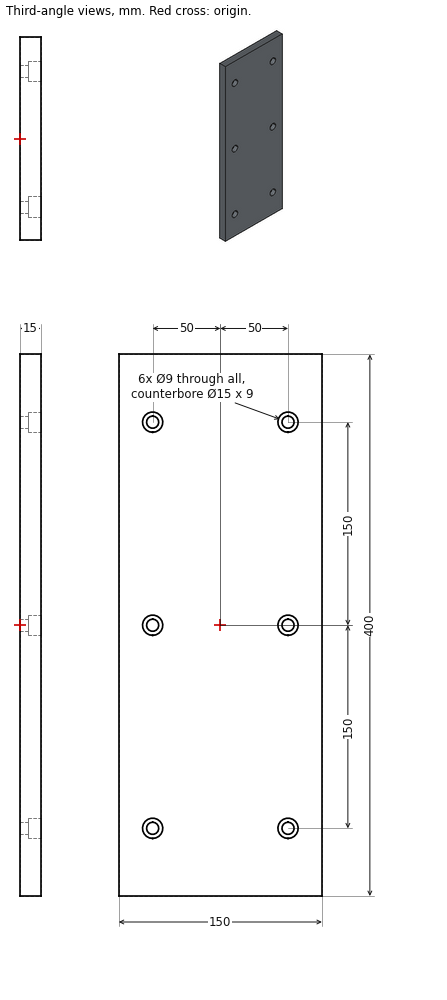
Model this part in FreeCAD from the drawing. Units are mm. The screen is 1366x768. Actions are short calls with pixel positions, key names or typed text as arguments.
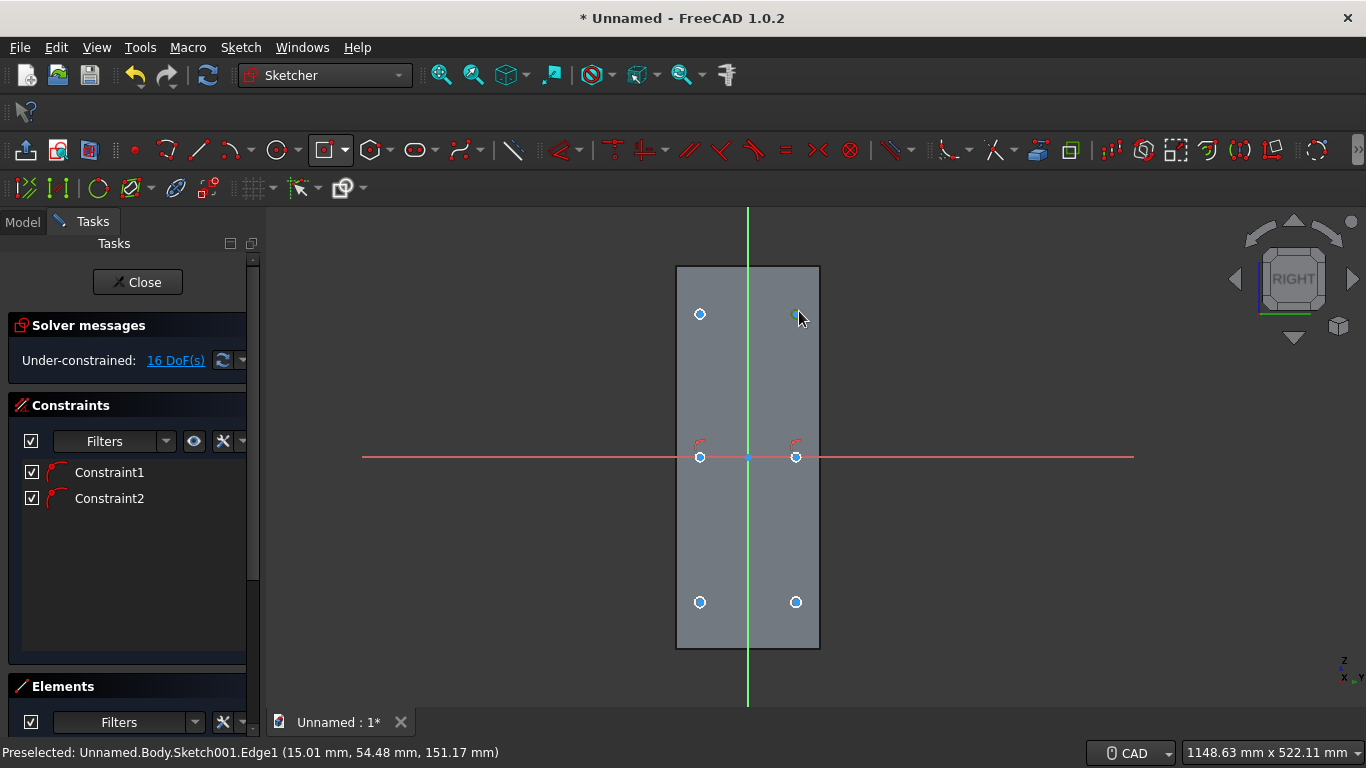
scroll(799, 454, up, 8)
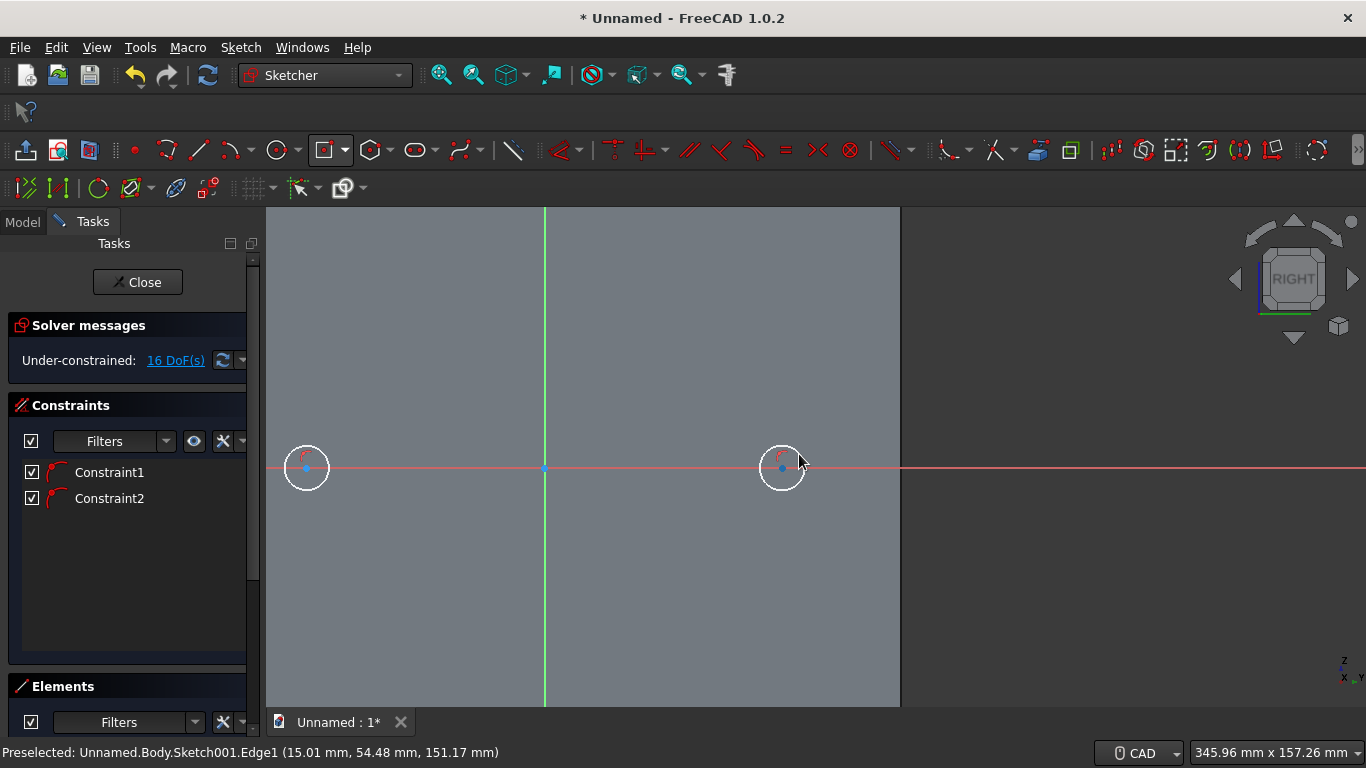
click(798, 452)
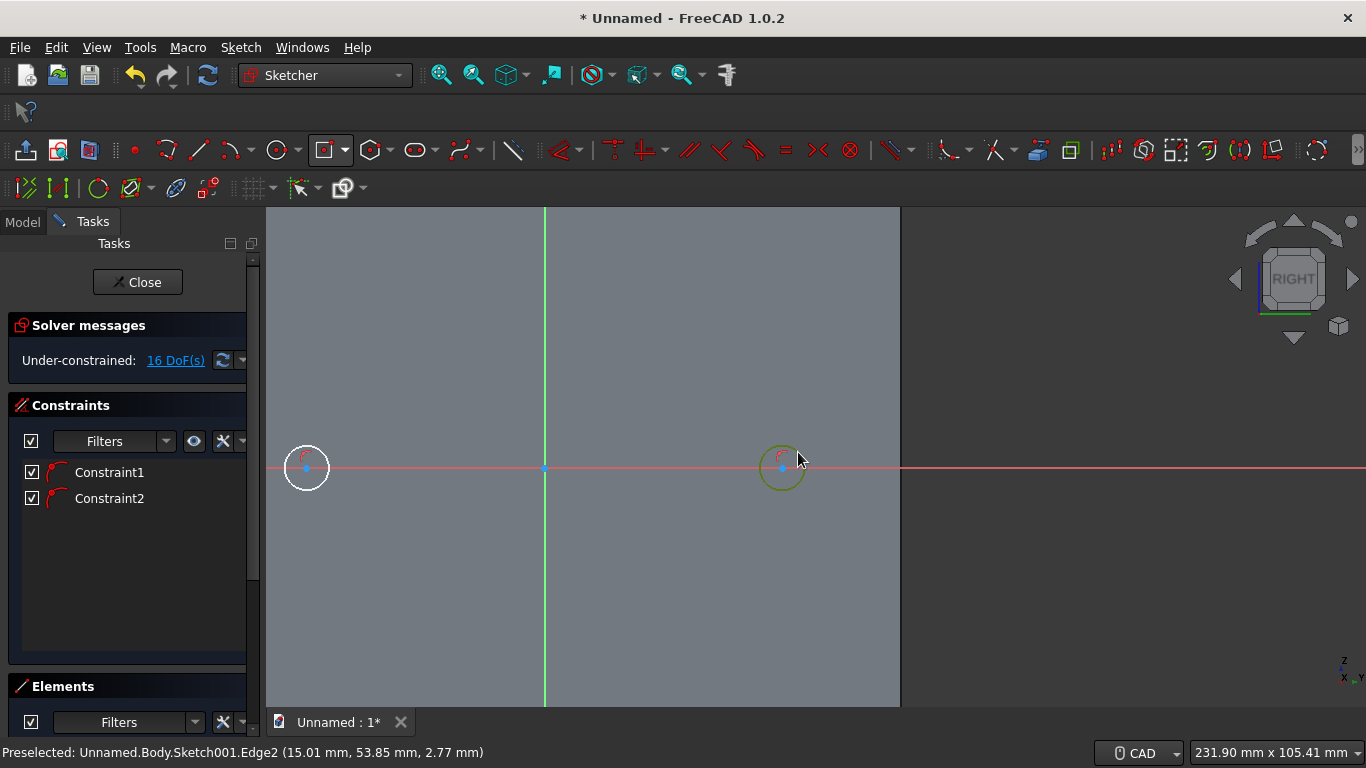
scroll(799, 454, down, 8)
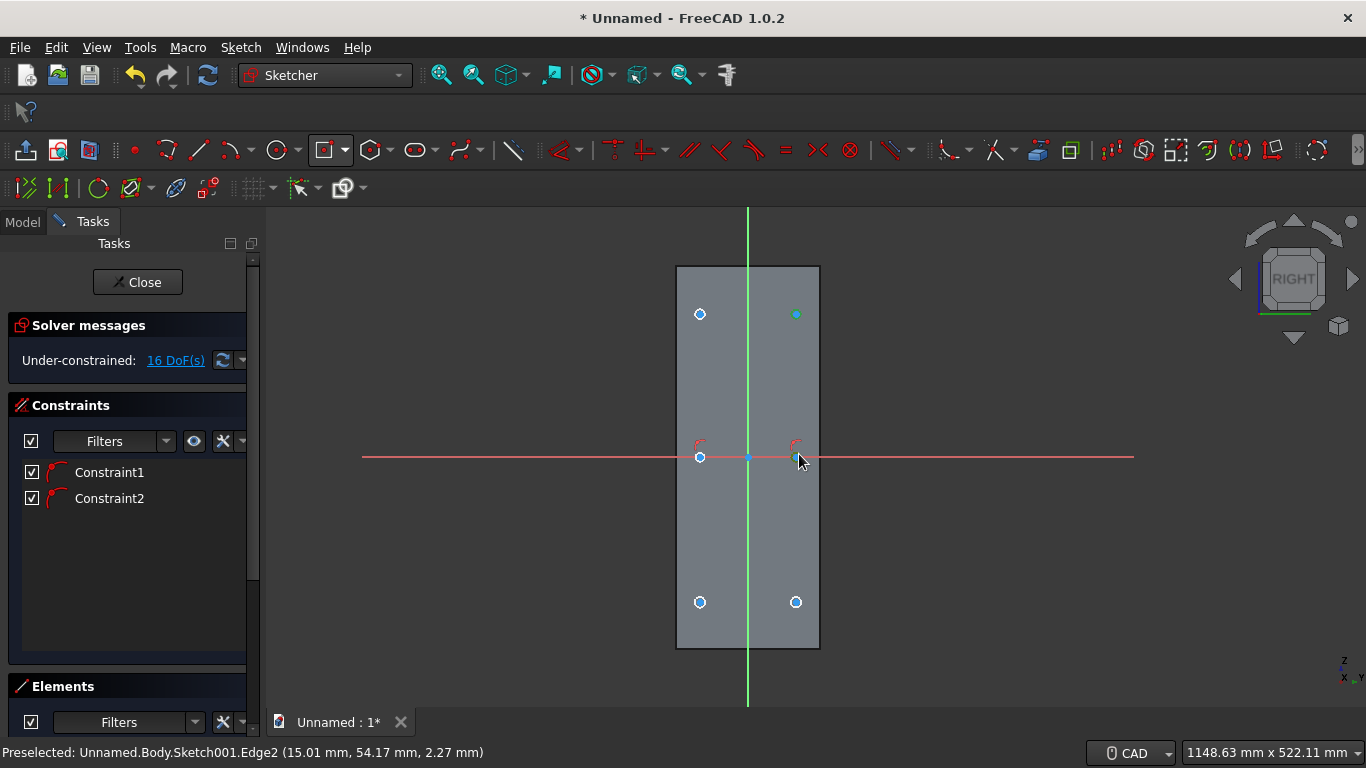
scroll(800, 599, up, 5)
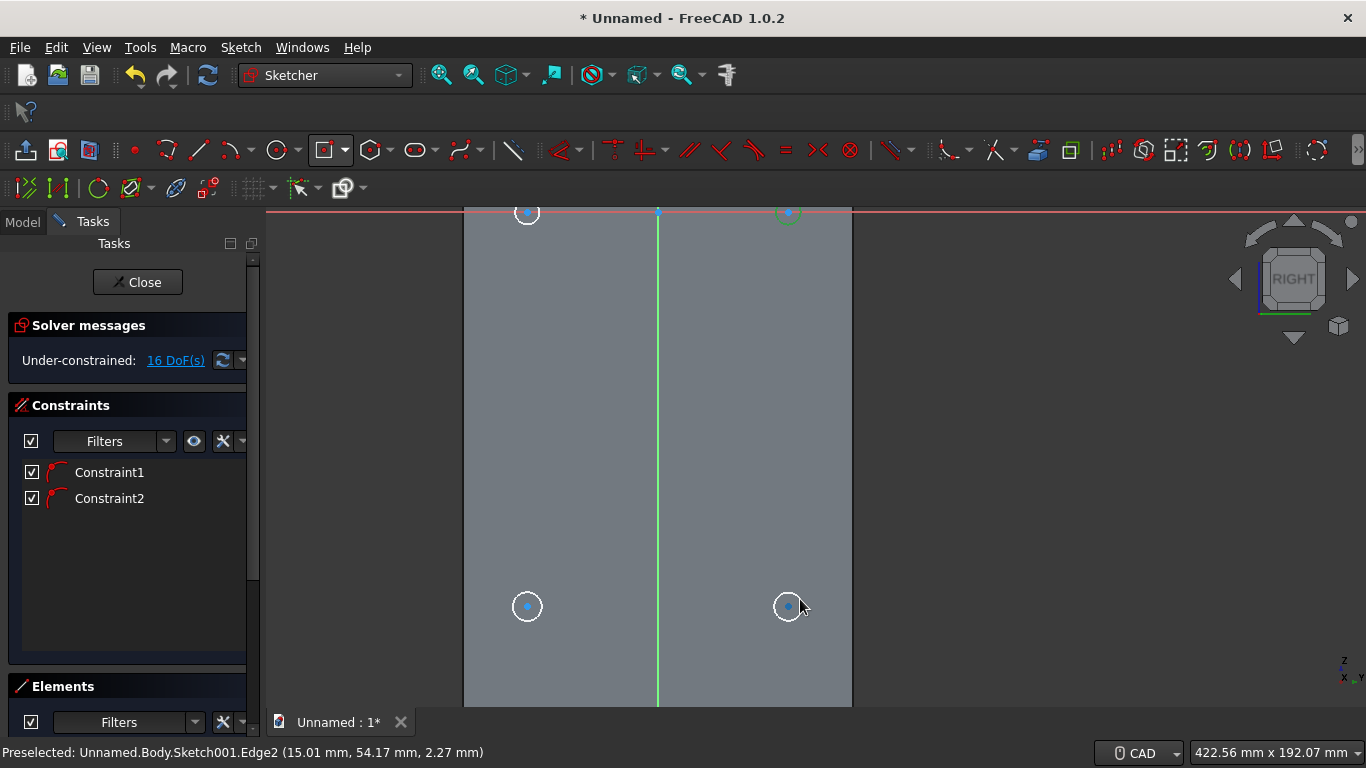
click(798, 597)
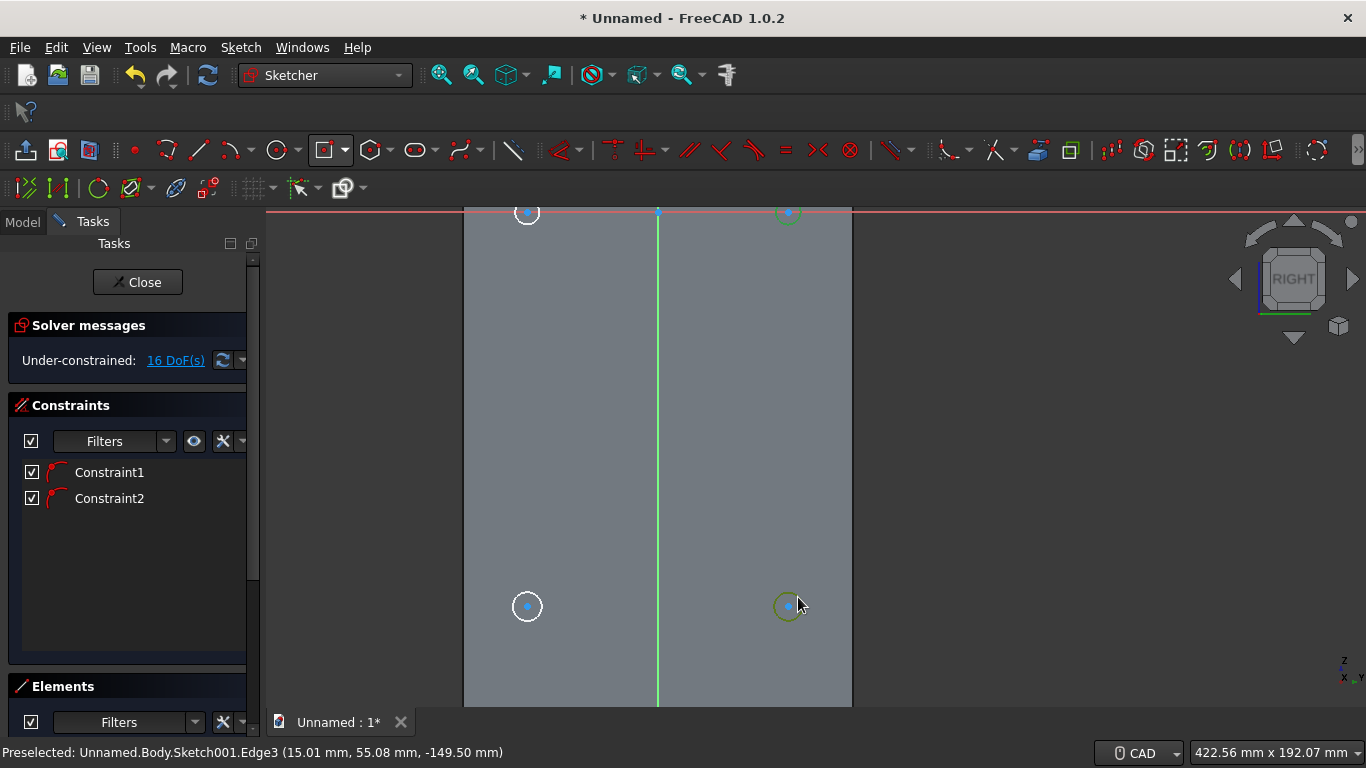
scroll(800, 599, down, 5)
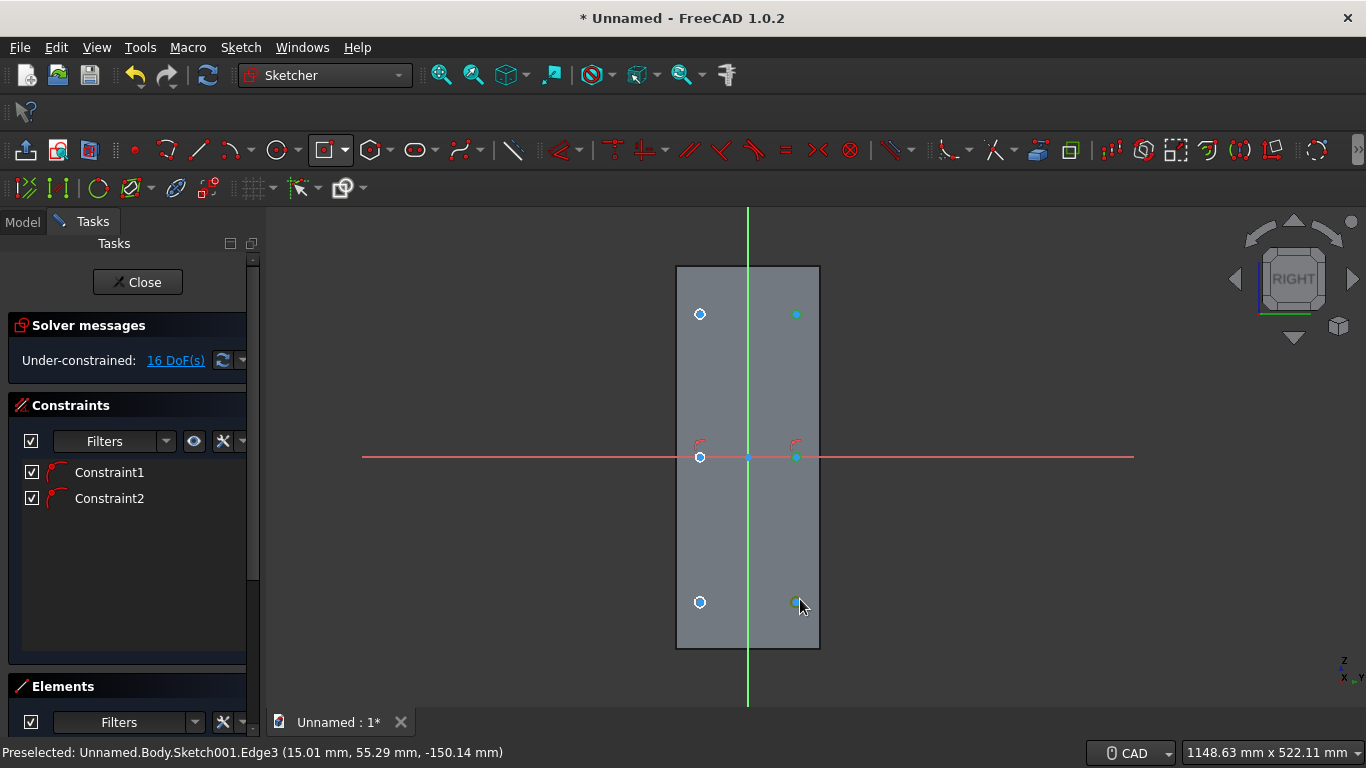
scroll(703, 311, up, 6)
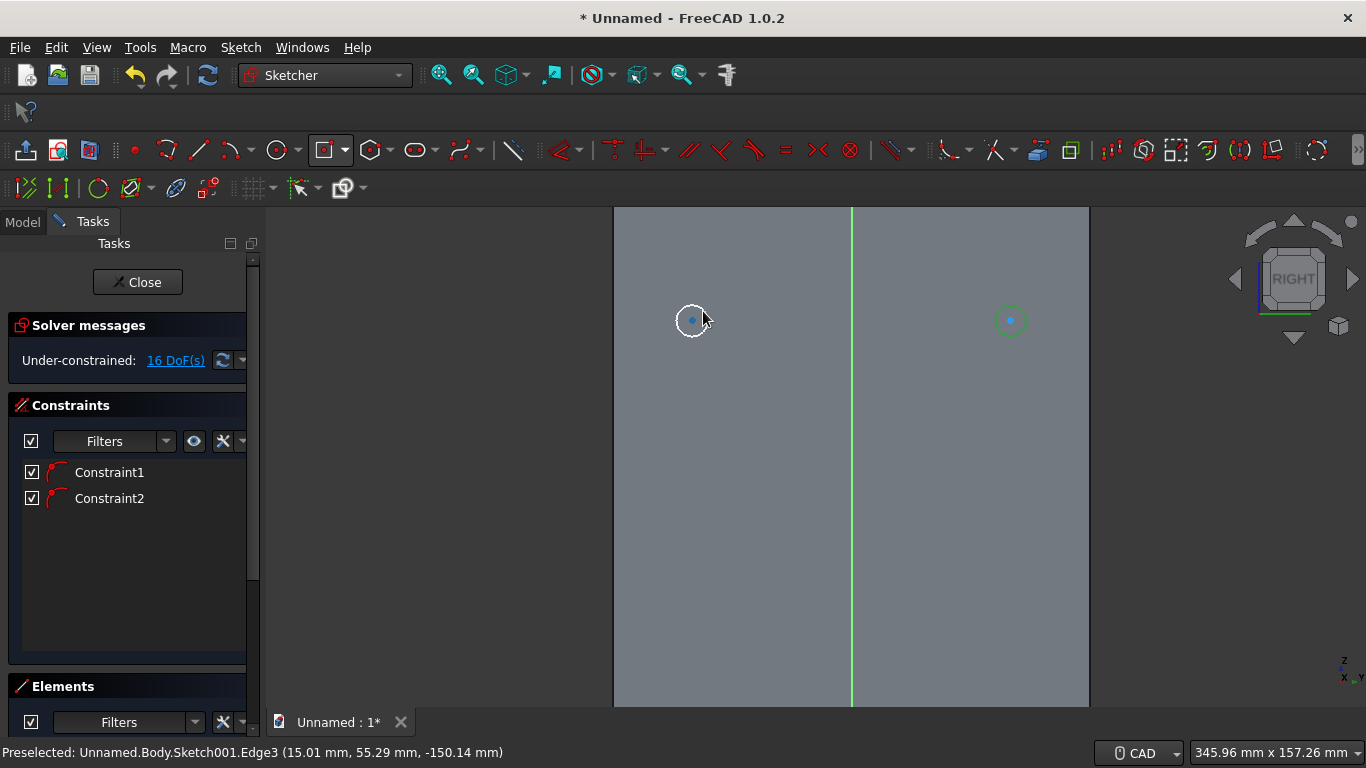
click(703, 310)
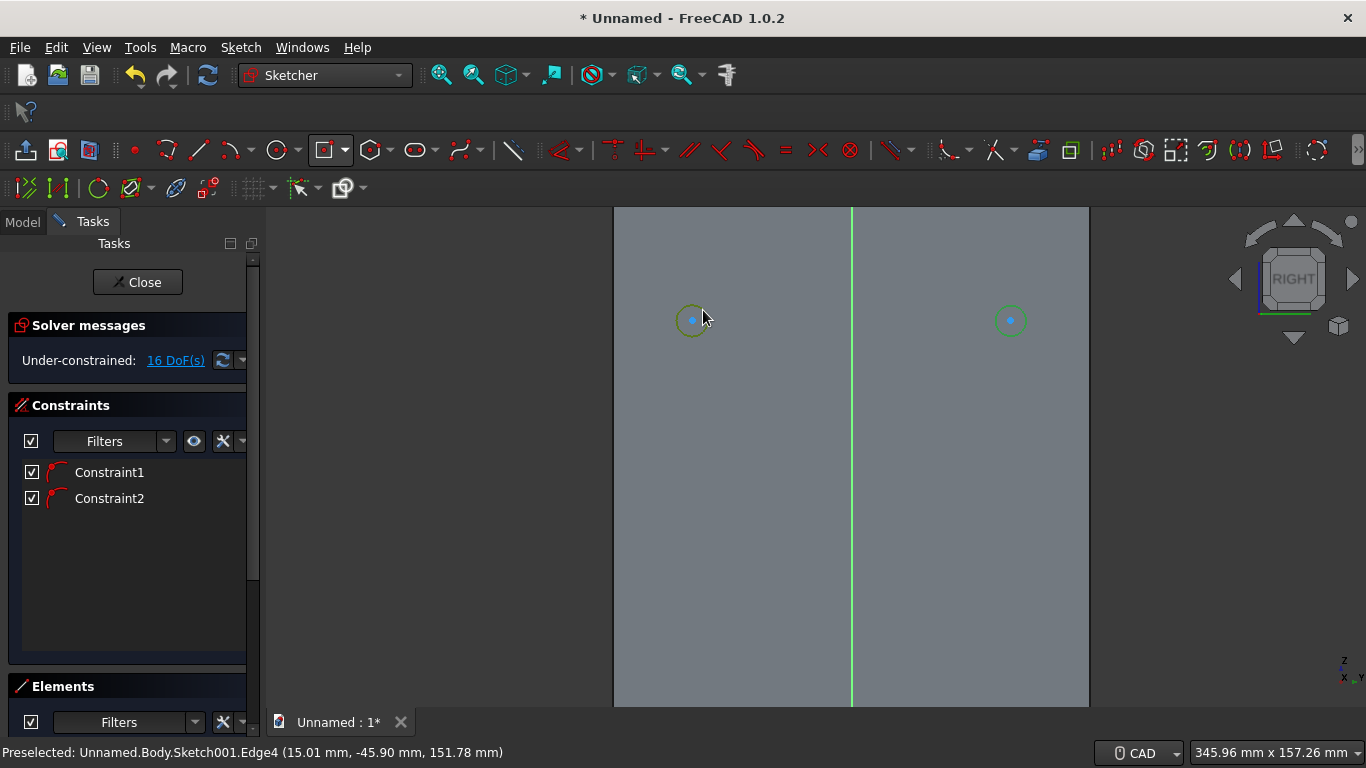
scroll(703, 311, down, 6)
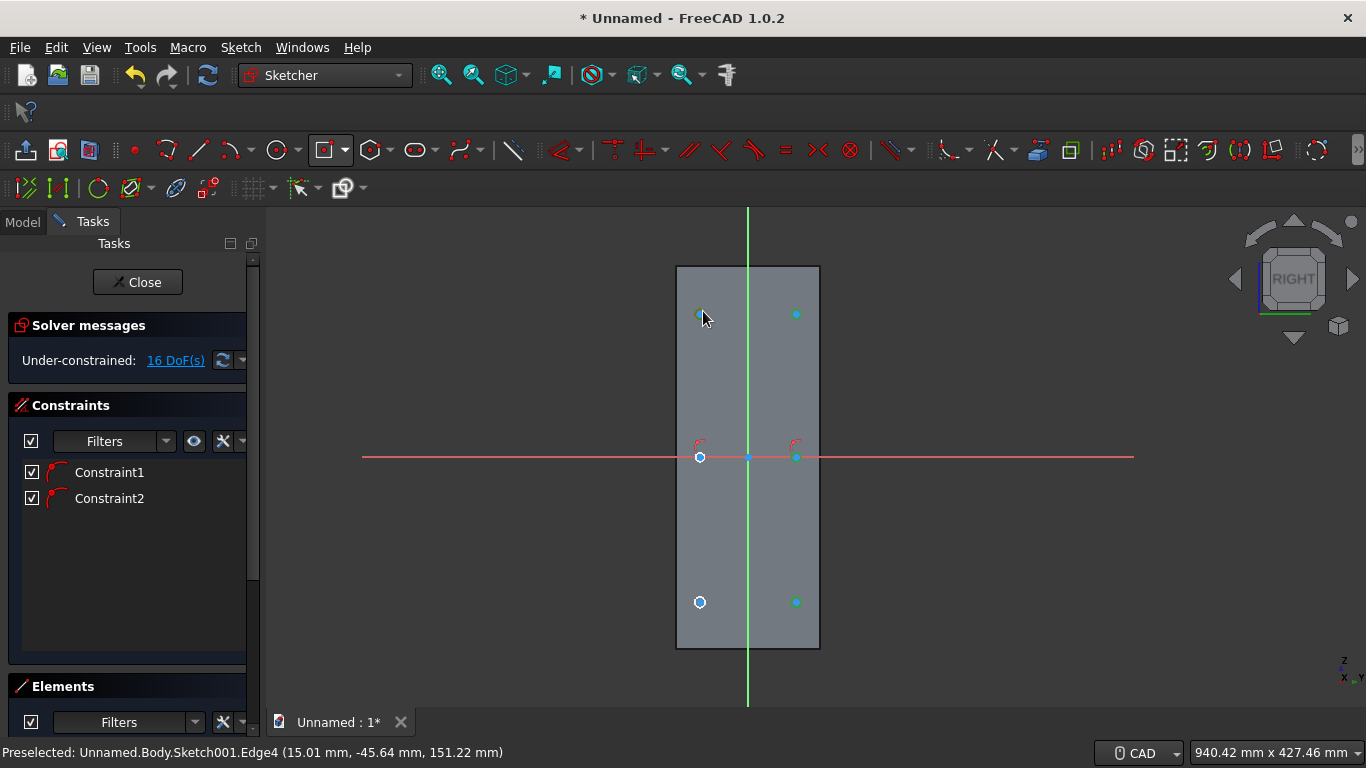
scroll(703, 454, up, 8)